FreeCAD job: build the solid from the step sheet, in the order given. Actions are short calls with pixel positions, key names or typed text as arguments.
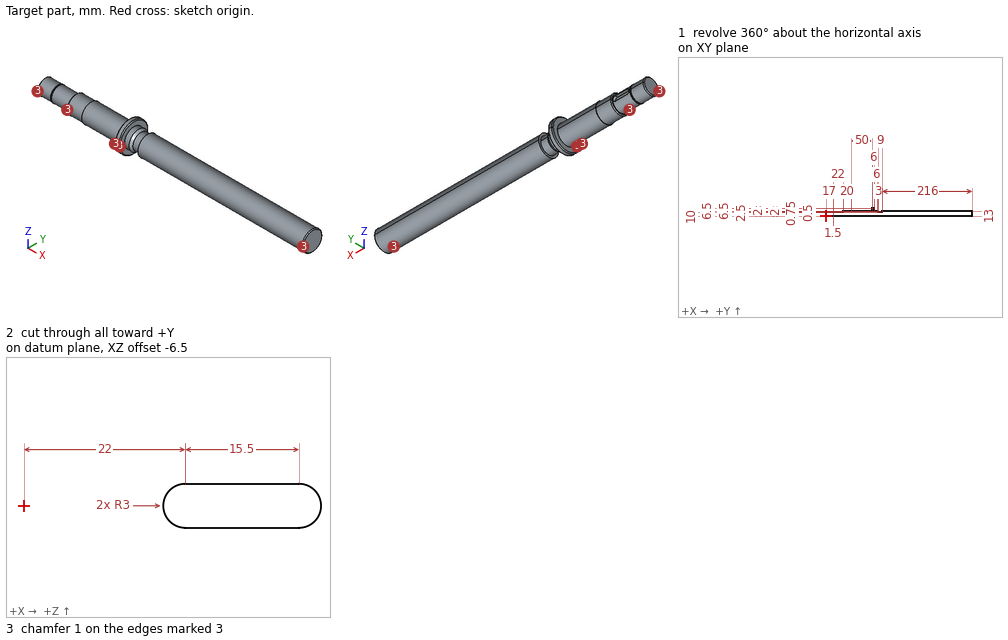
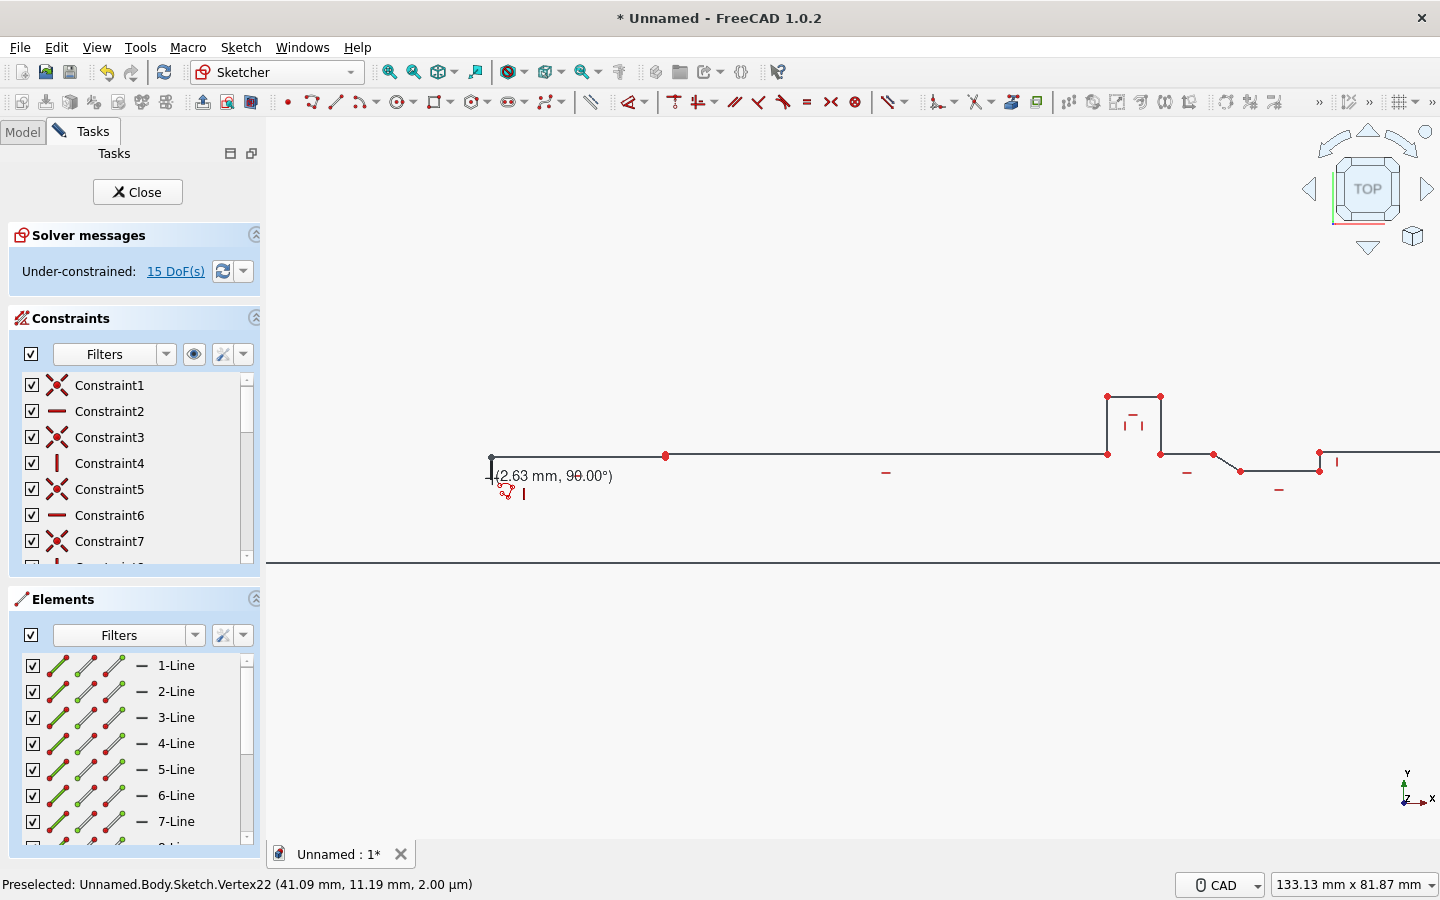
click(491, 475)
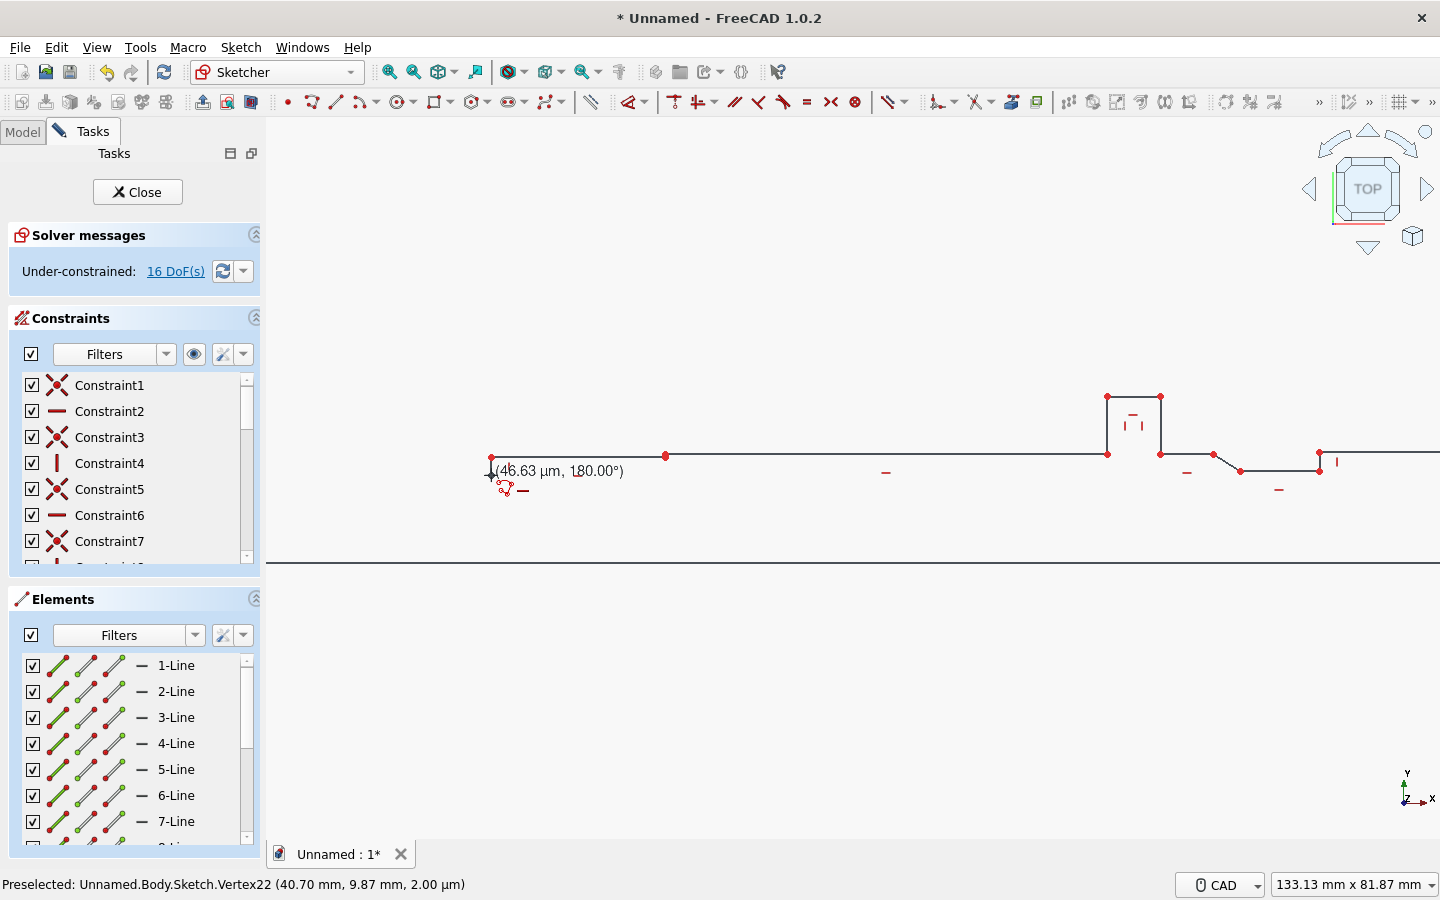
scroll(492, 478, down, 7)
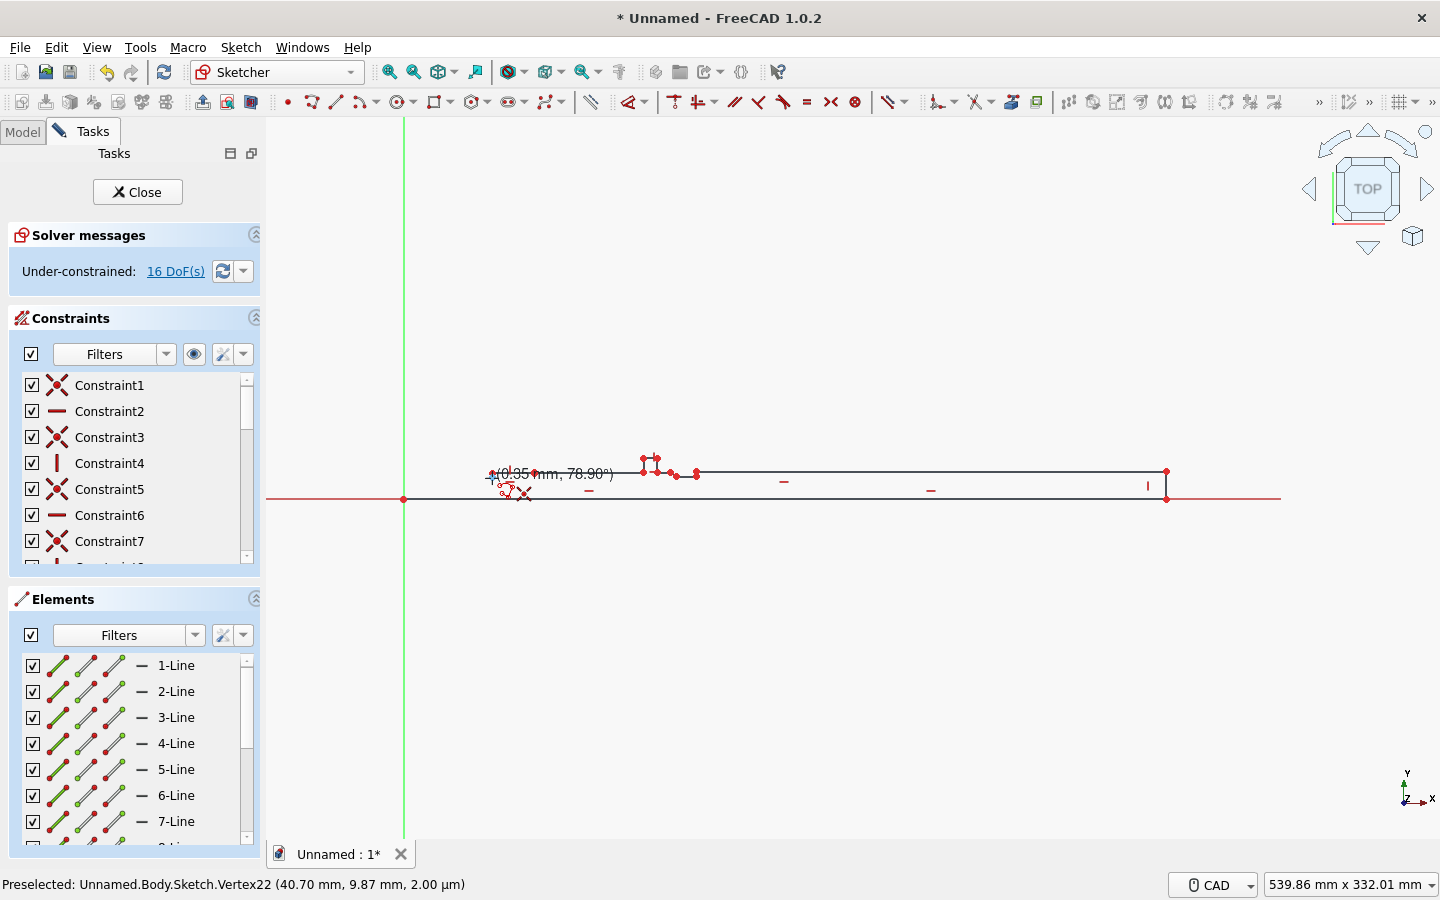
click(444, 478)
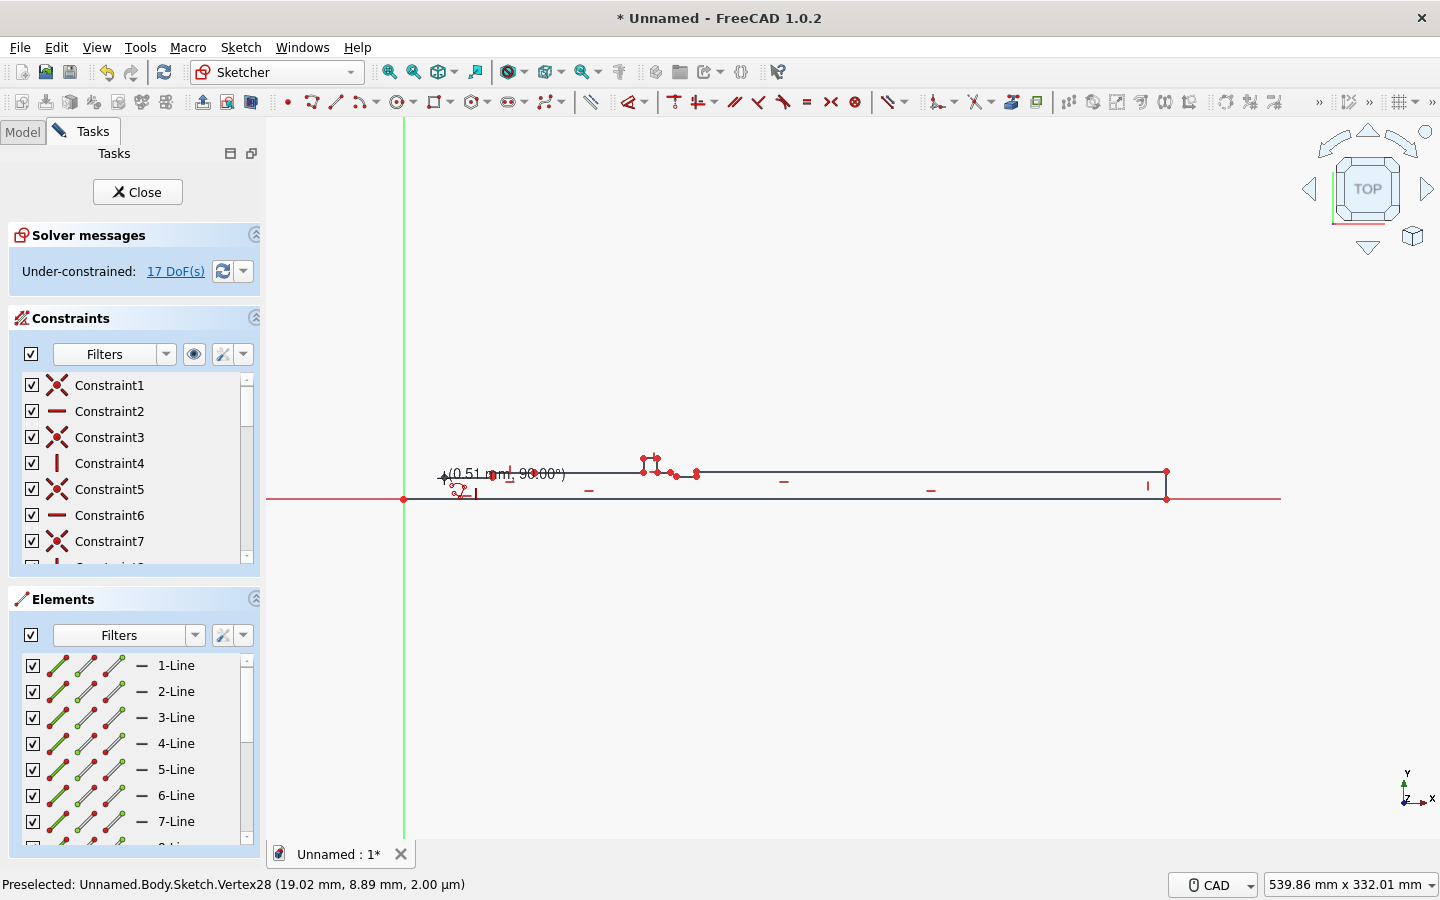
scroll(444, 479, up, 12)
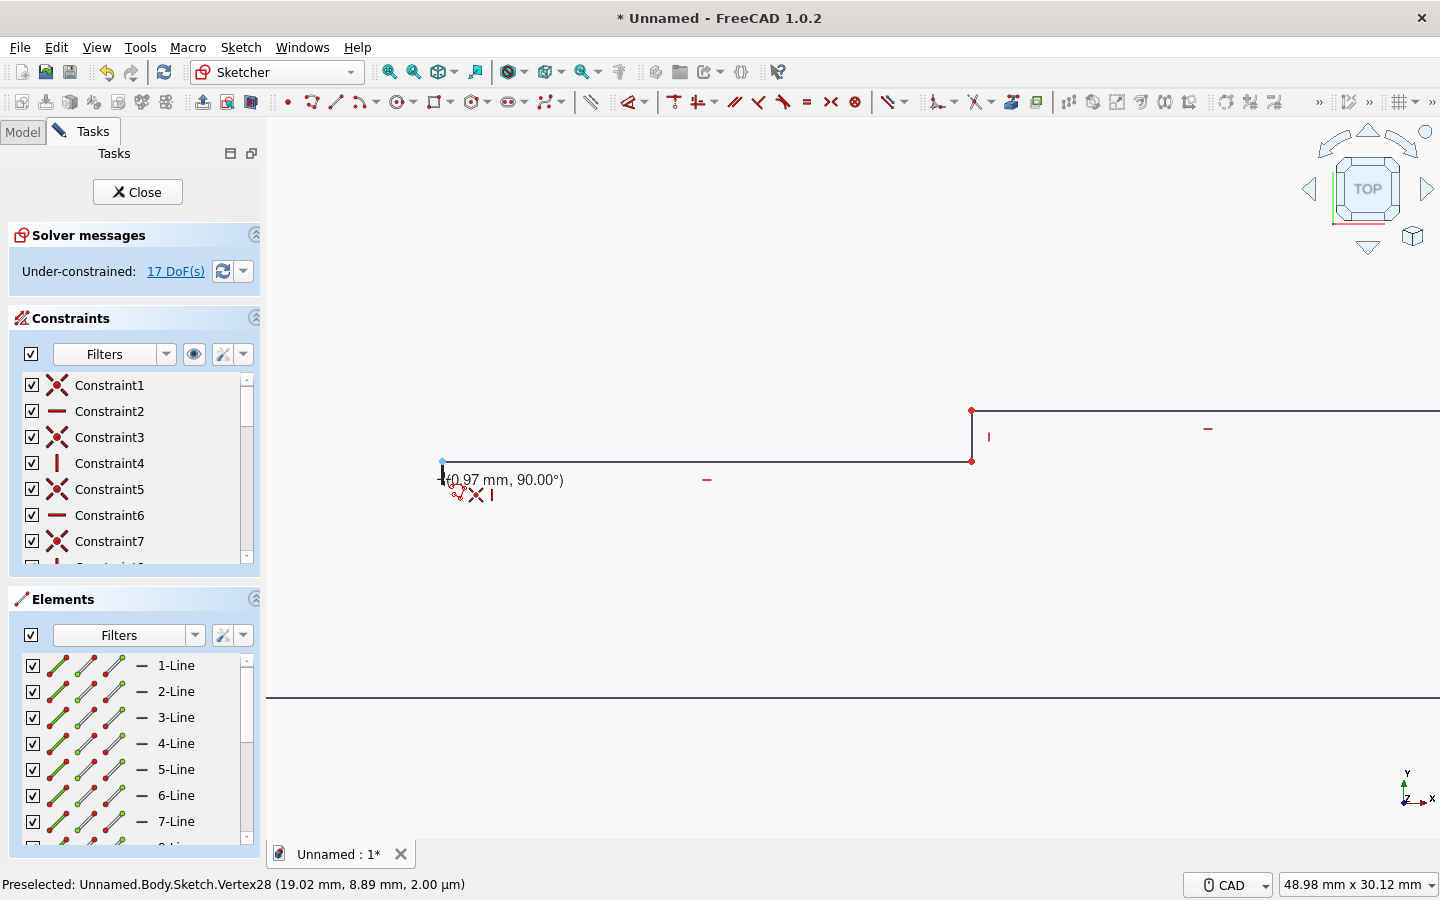
click(442, 476)
click(405, 476)
click(405, 459)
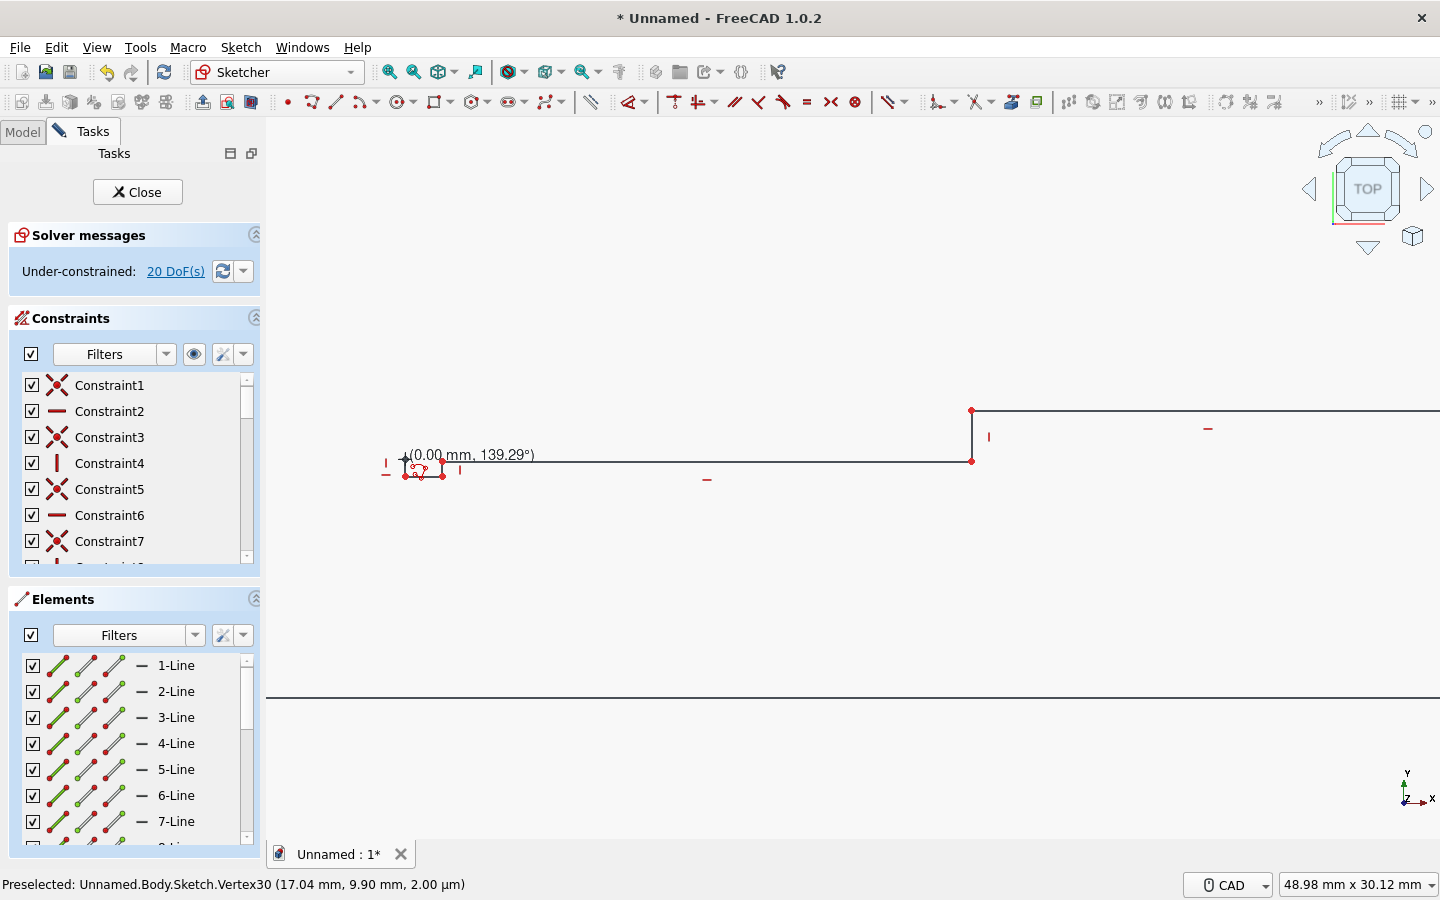
scroll(444, 479, down, 12)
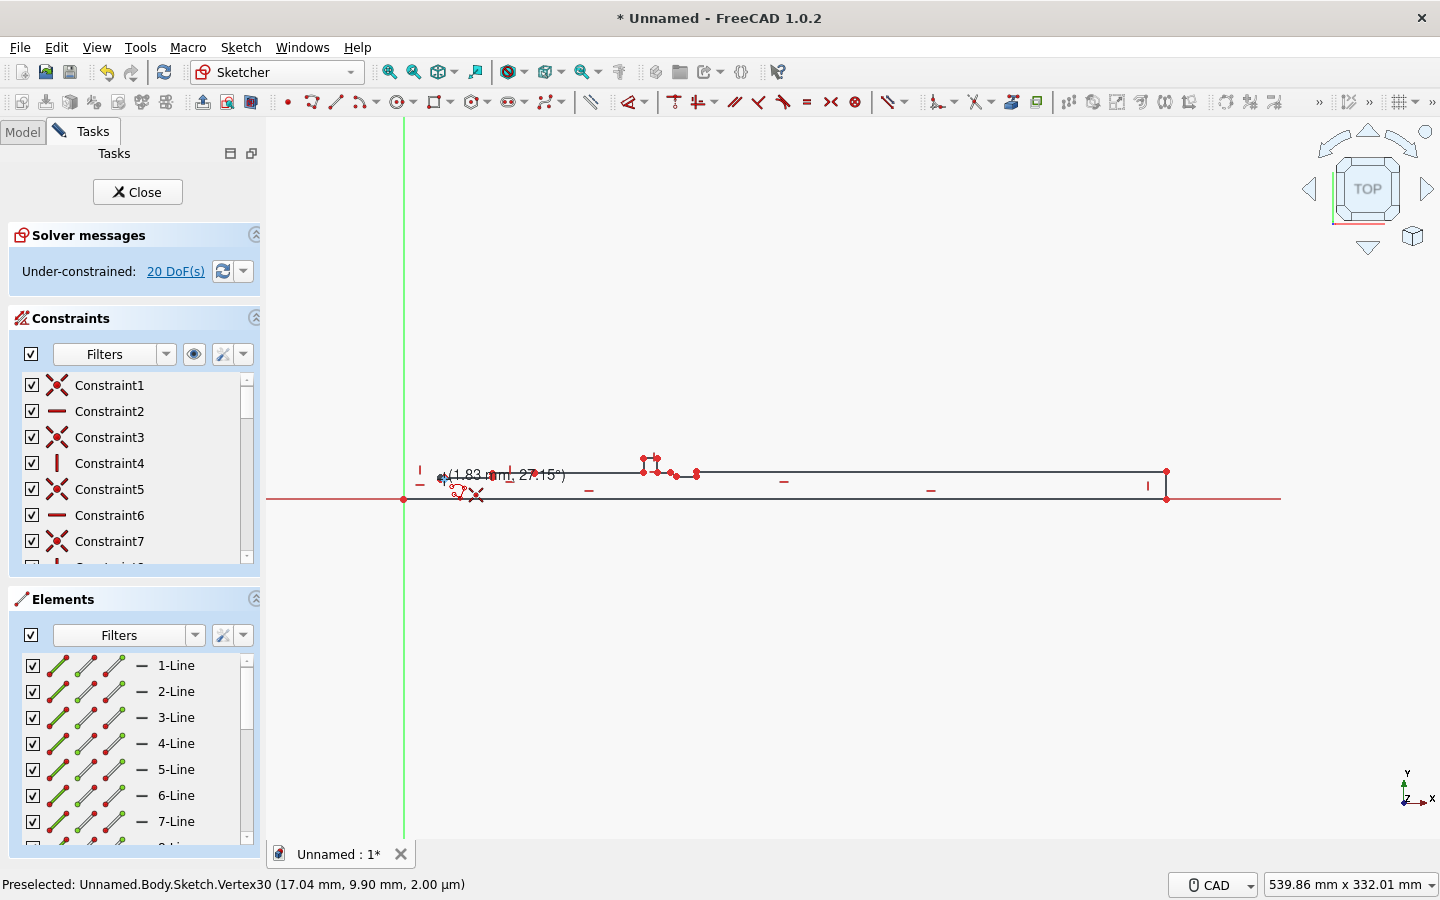
click(413, 478)
click(404, 499)
key(Escape)
key(Escape)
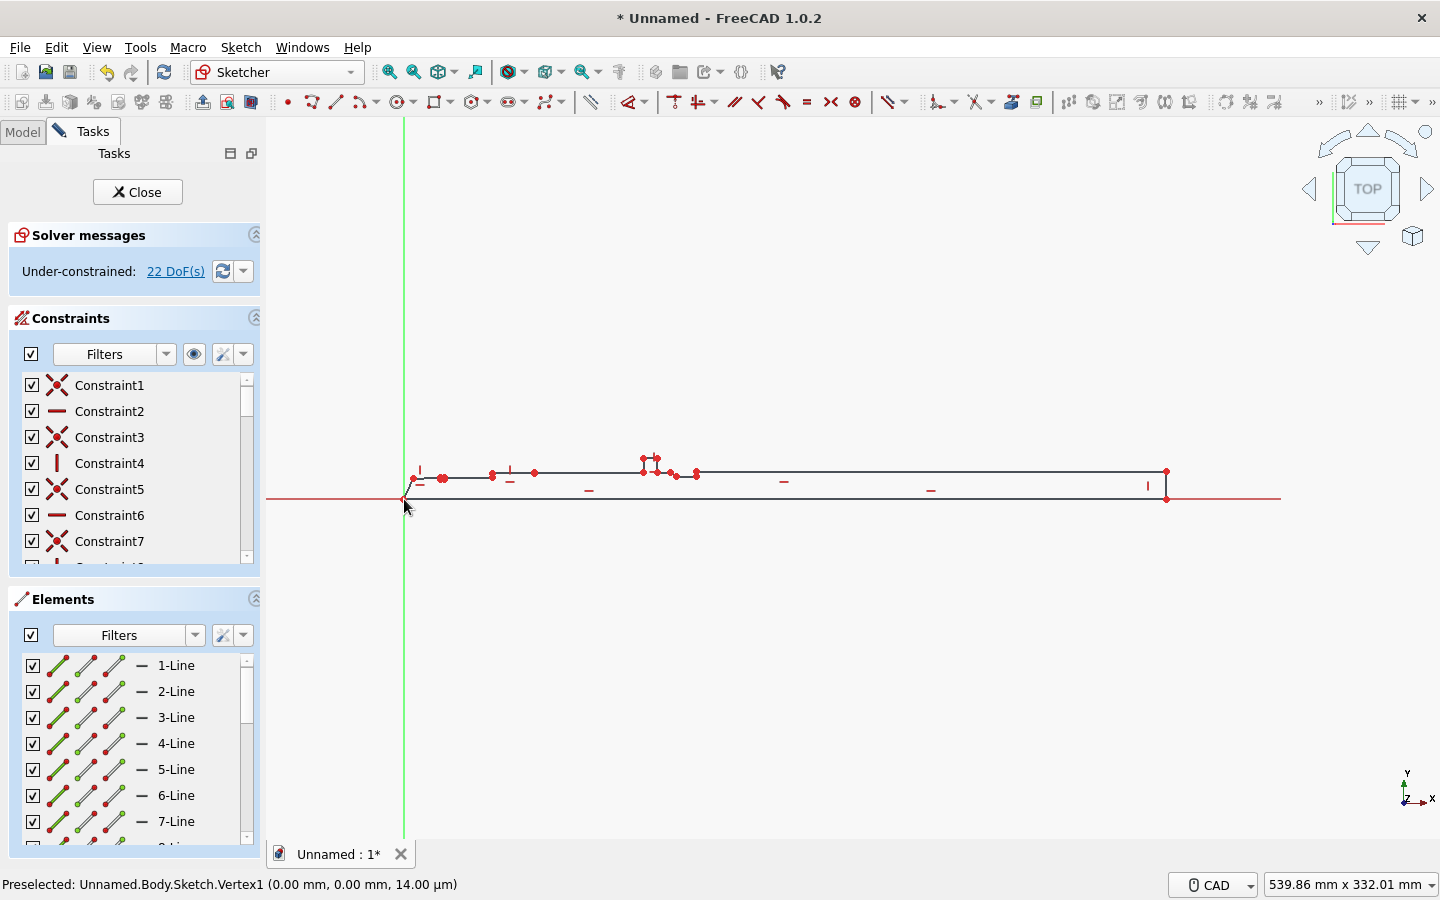
scroll(535, 473, up, 14)